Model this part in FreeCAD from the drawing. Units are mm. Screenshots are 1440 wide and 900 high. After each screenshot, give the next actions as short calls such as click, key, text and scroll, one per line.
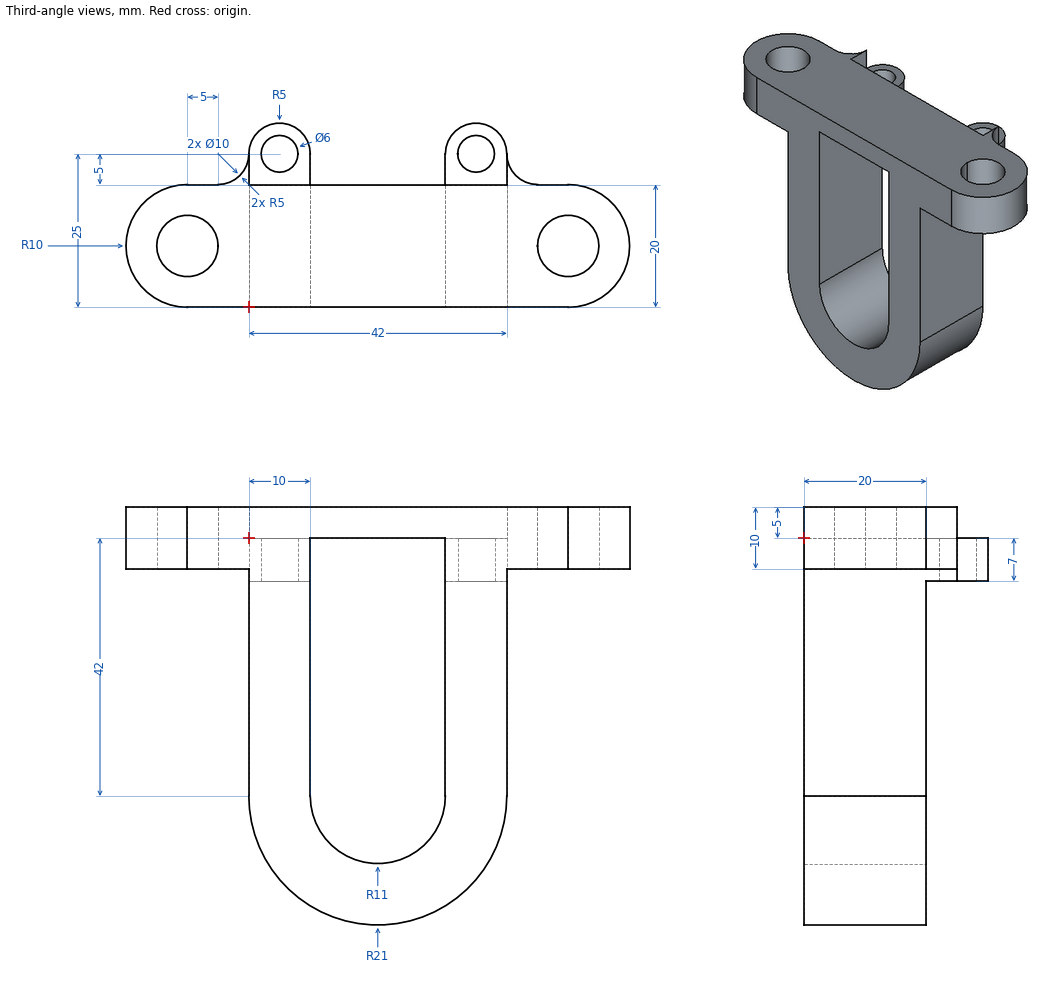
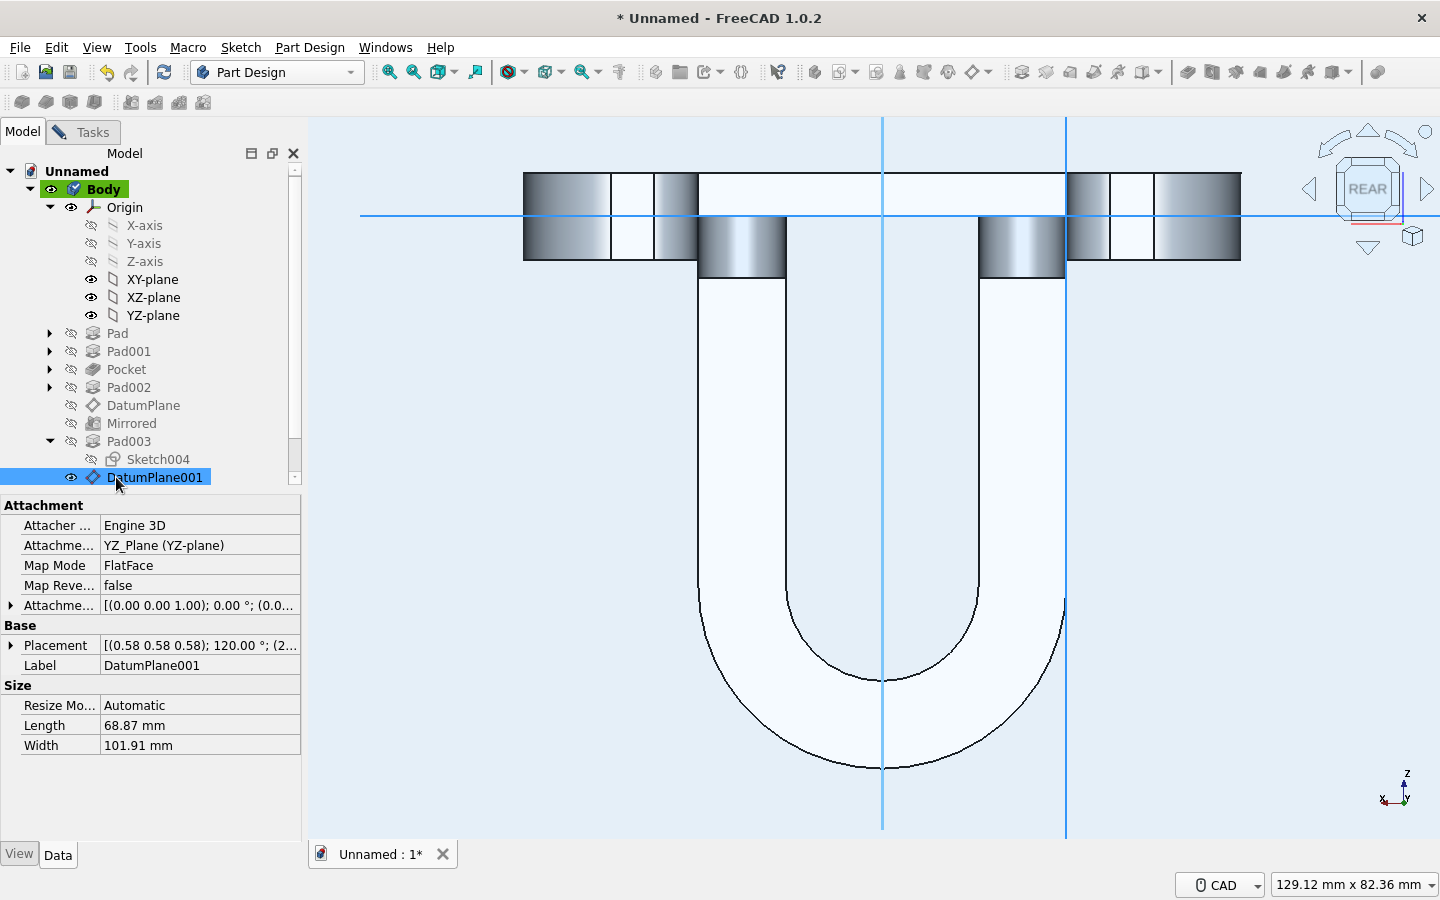
click(84, 131)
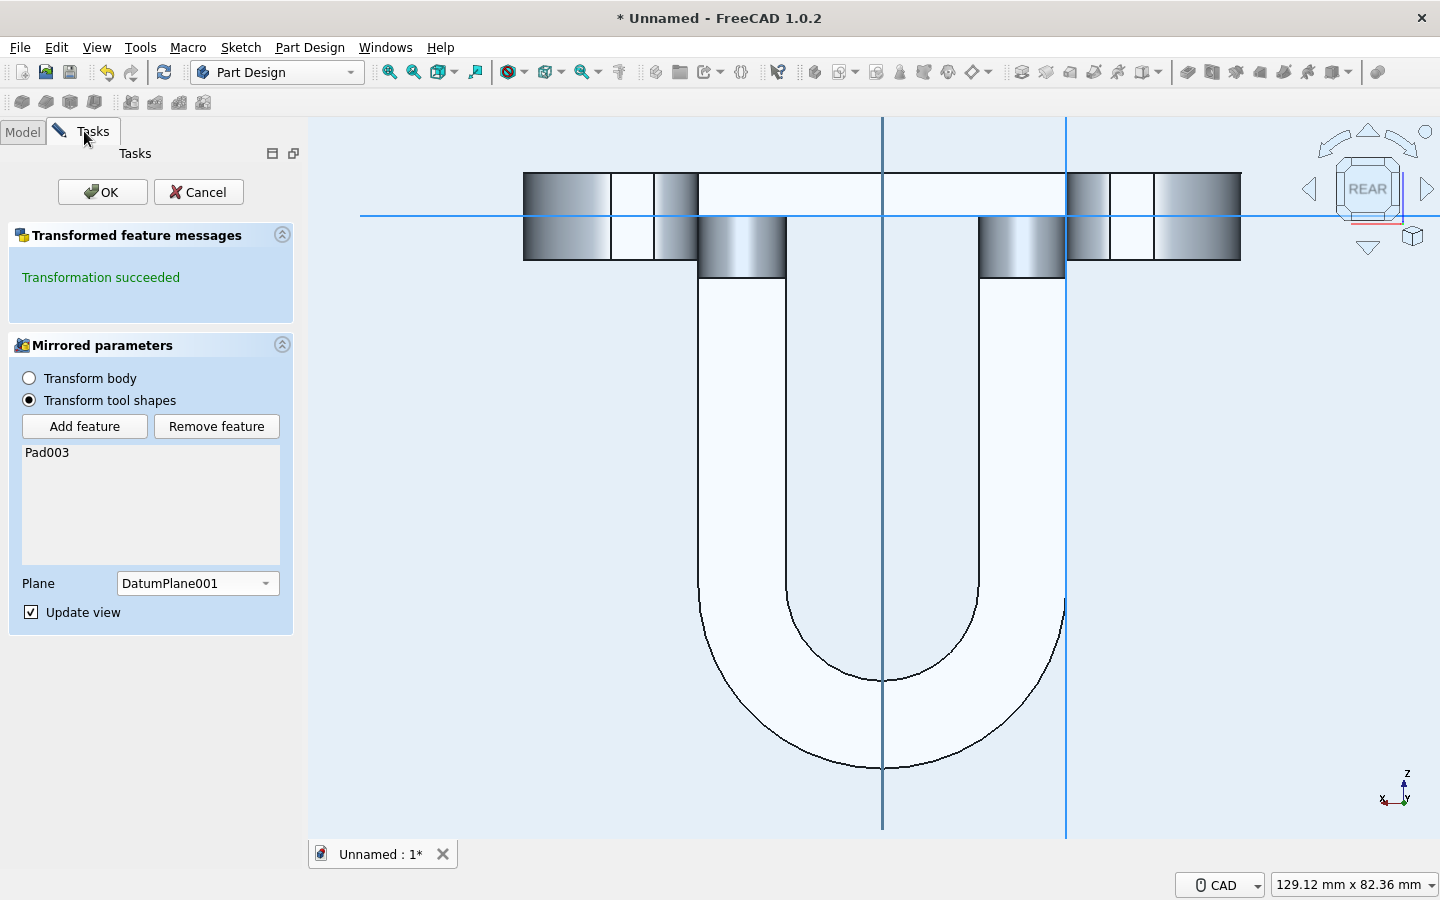
click(103, 192)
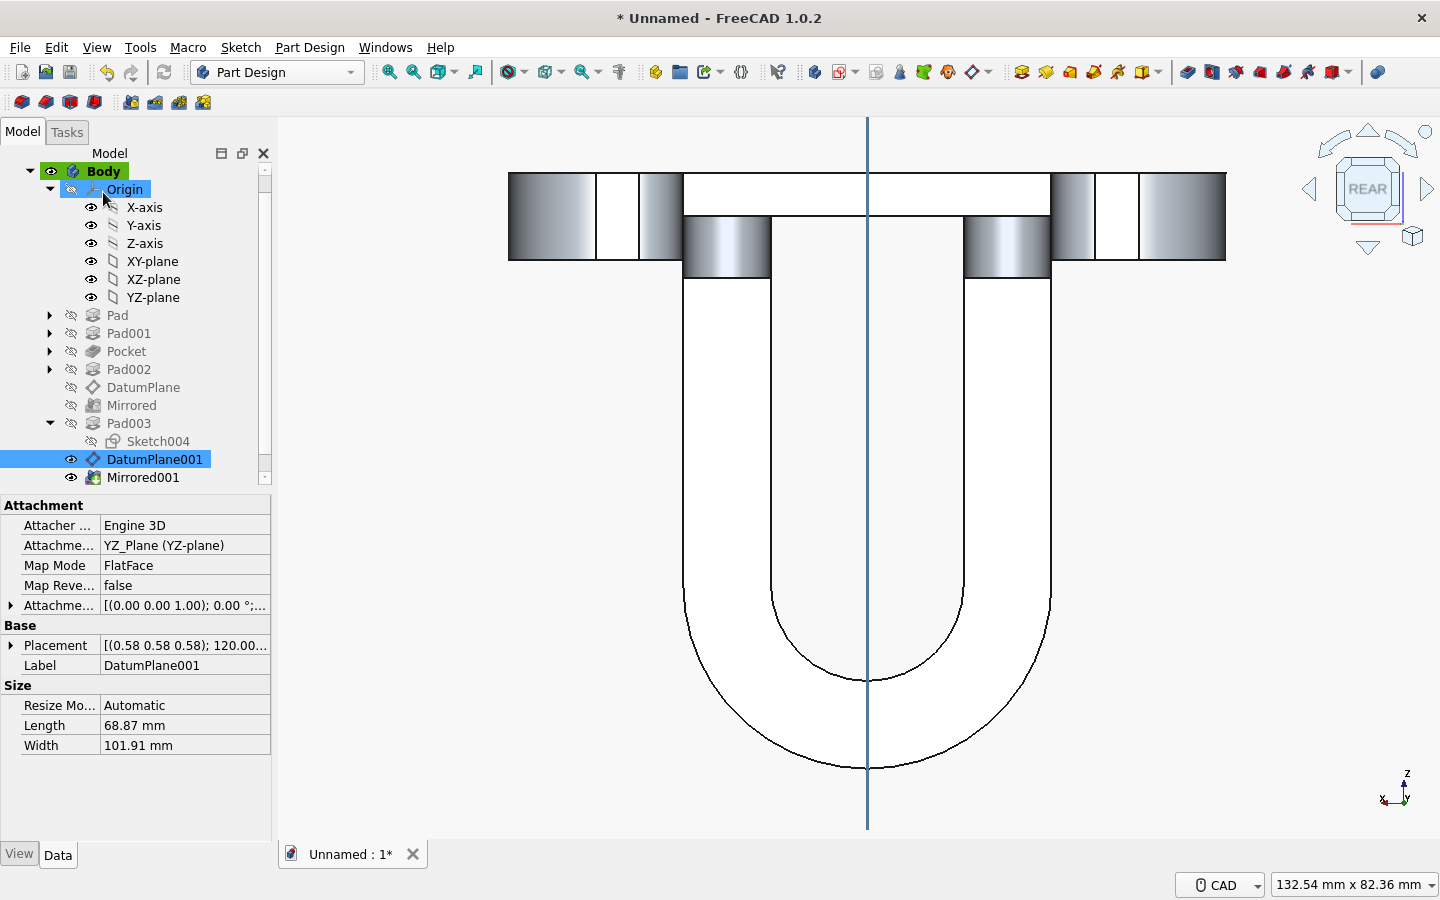
click(116, 459)
key(space)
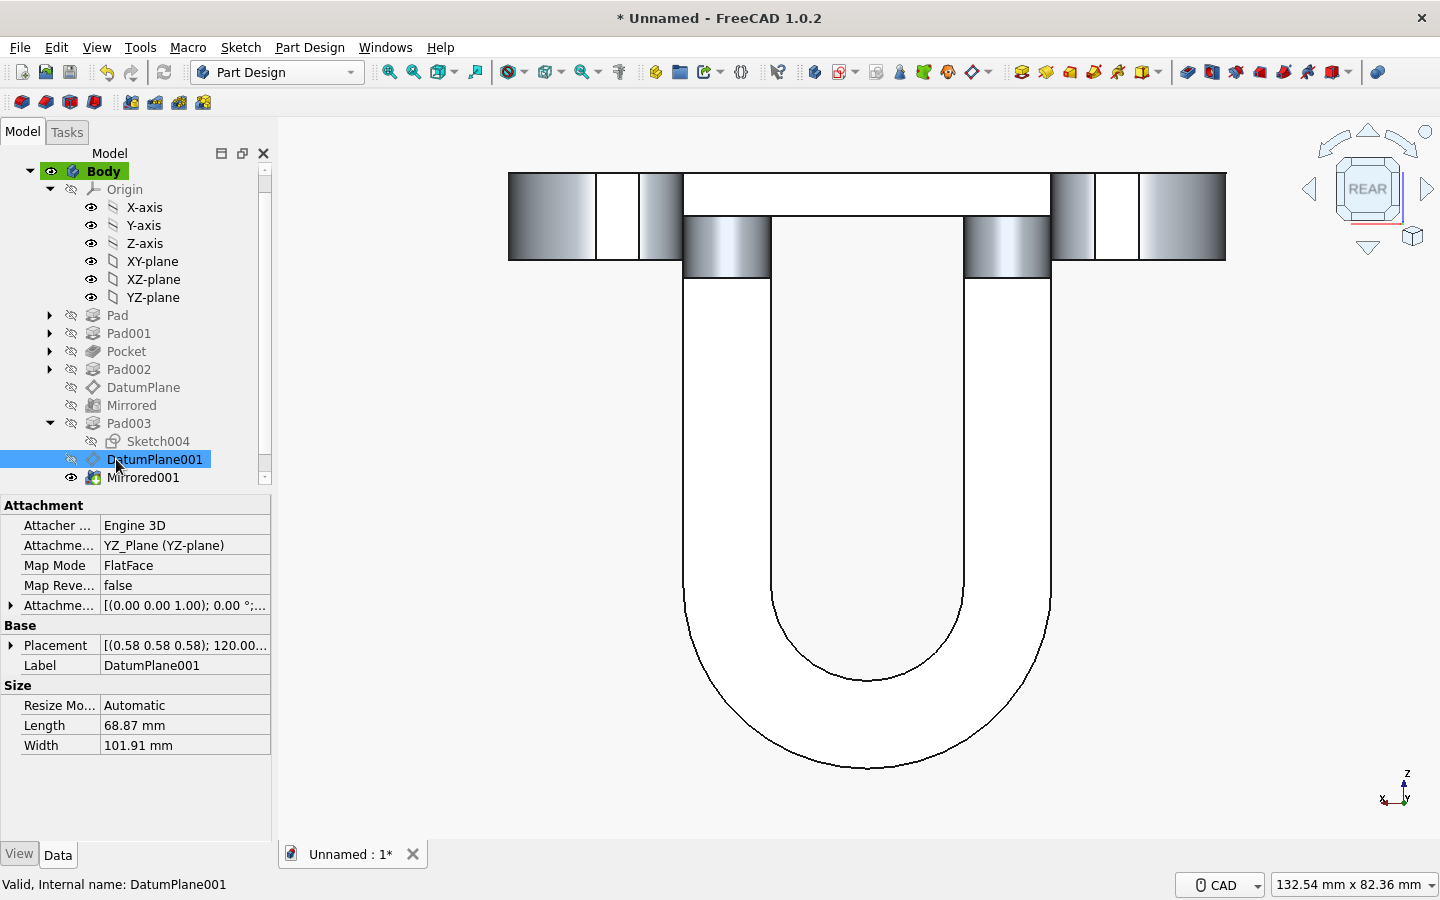
key(0)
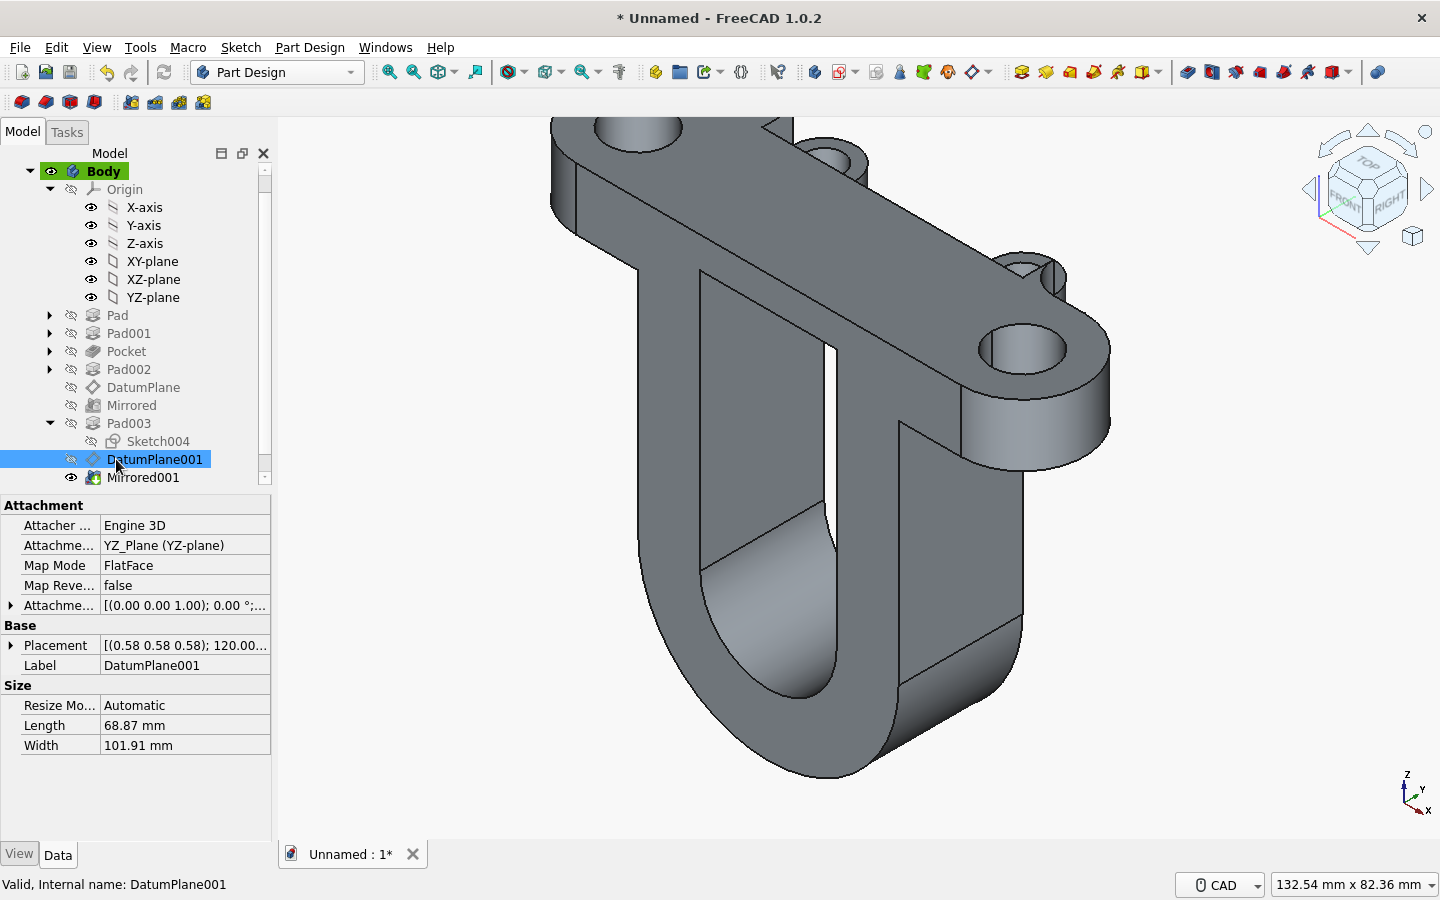
click(390, 72)